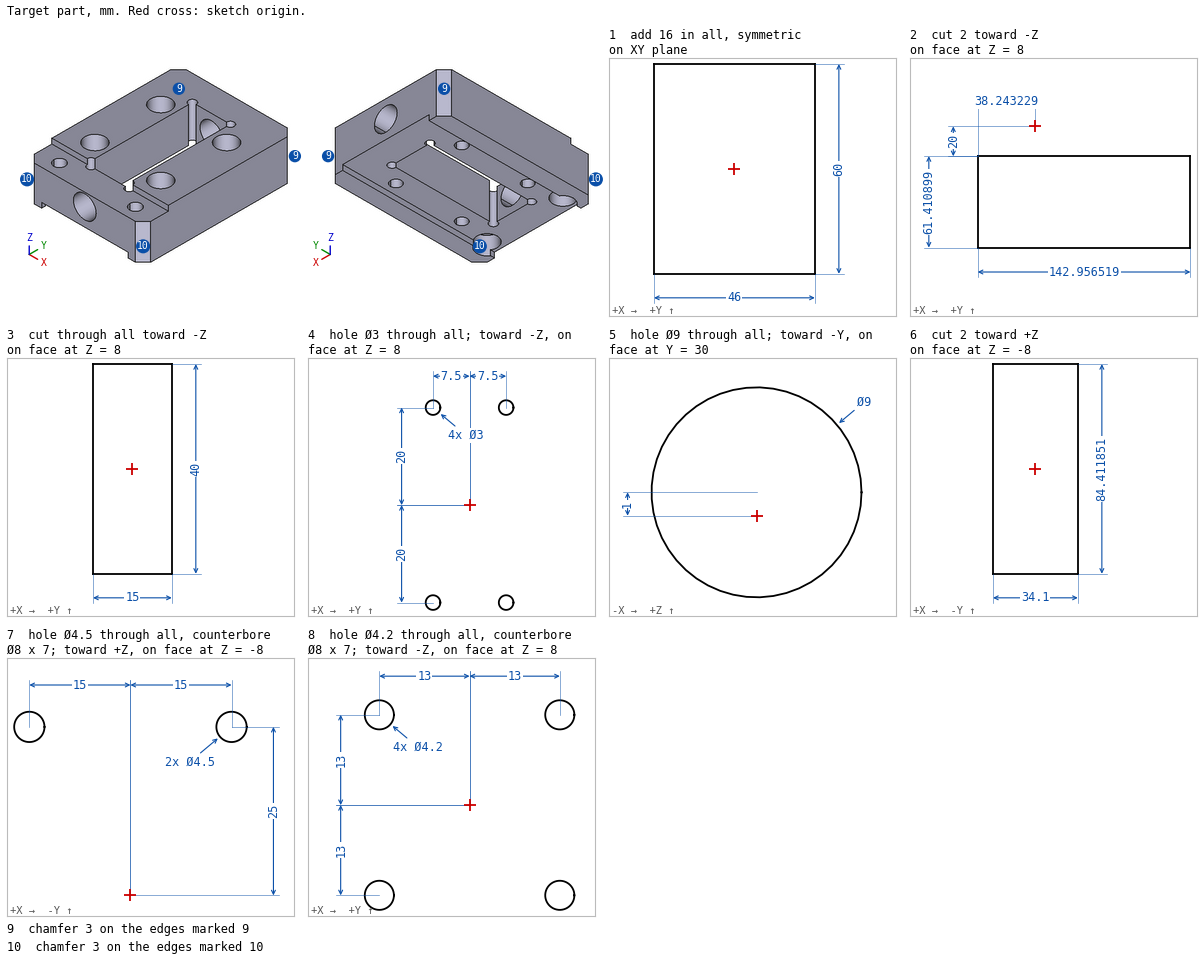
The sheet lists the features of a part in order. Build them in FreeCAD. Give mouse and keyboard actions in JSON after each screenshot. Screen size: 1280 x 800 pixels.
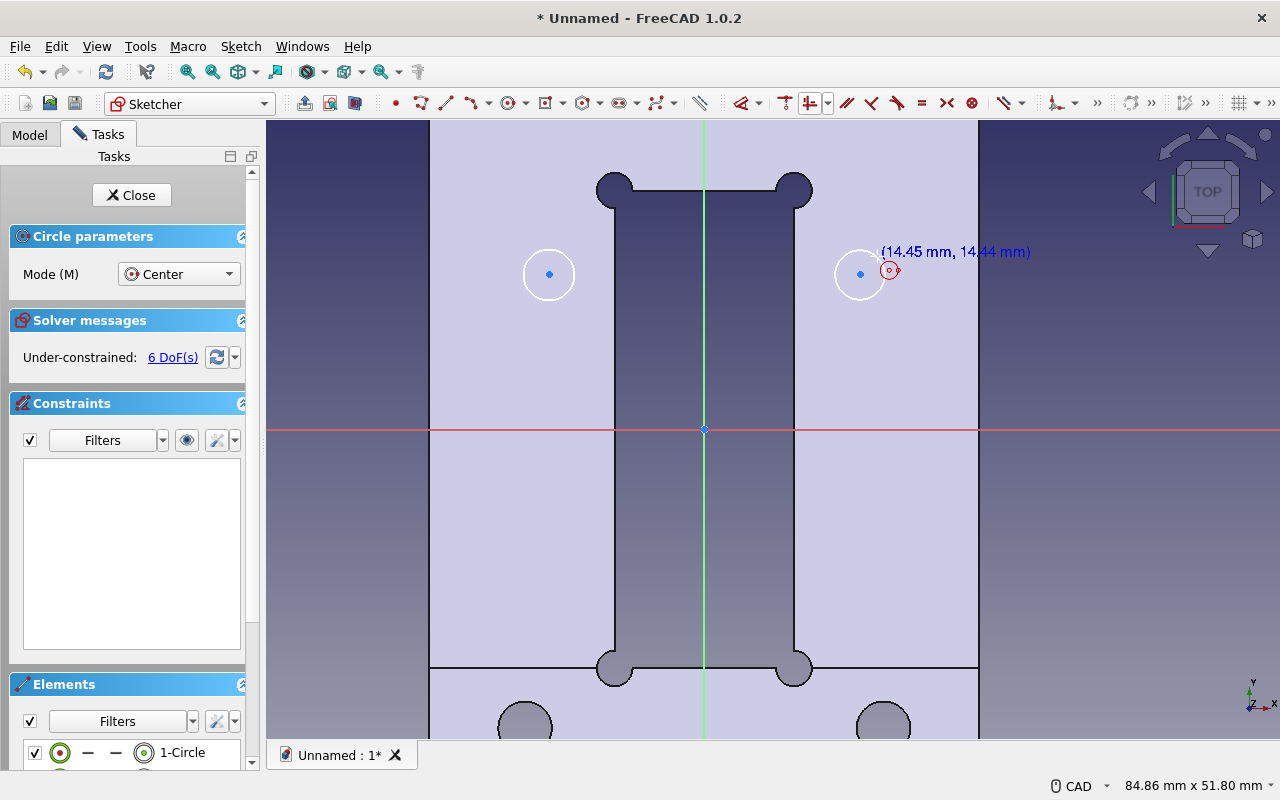
{"action": "left_click", "coordinate": [549, 585]}
{"action": "left_click", "coordinate": [567, 567]}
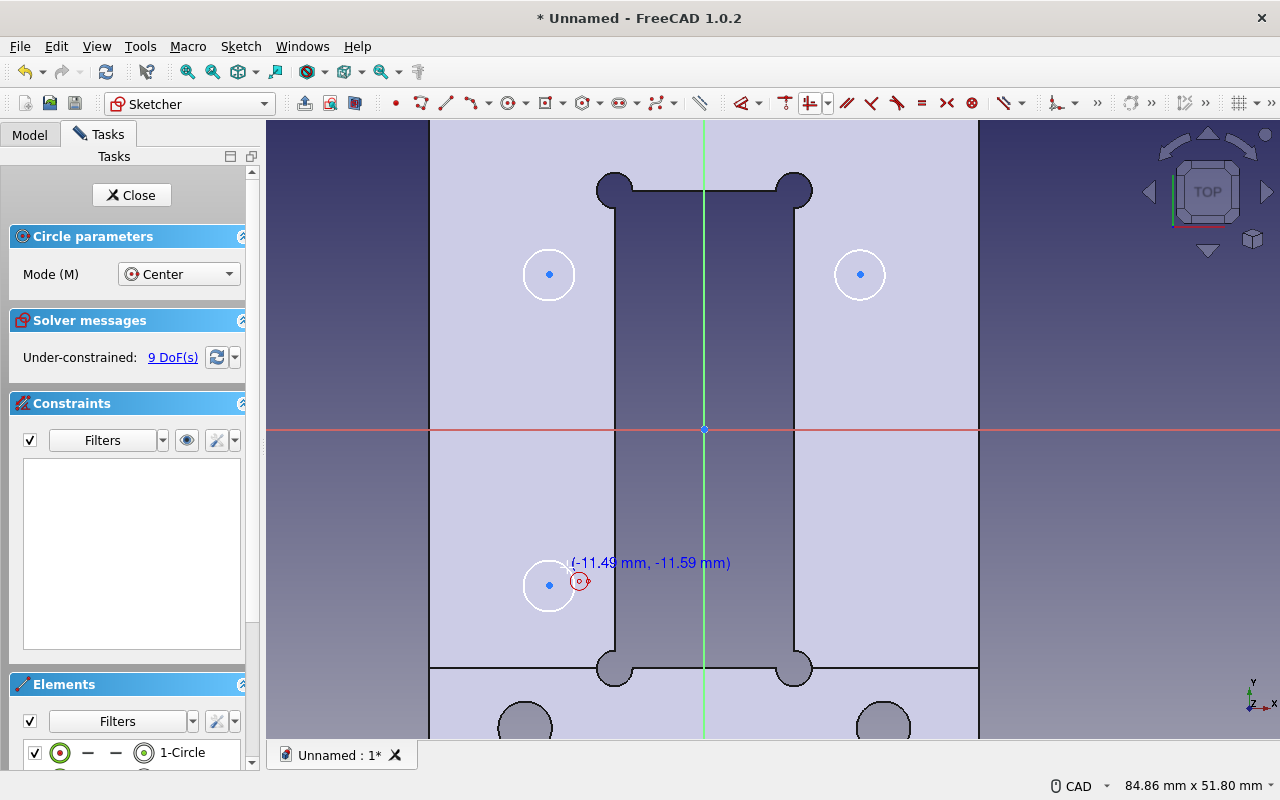
{"action": "left_click", "coordinate": [860, 585]}
{"action": "left_click", "coordinate": [877, 567]}
{"action": "key", "text": "Escape"}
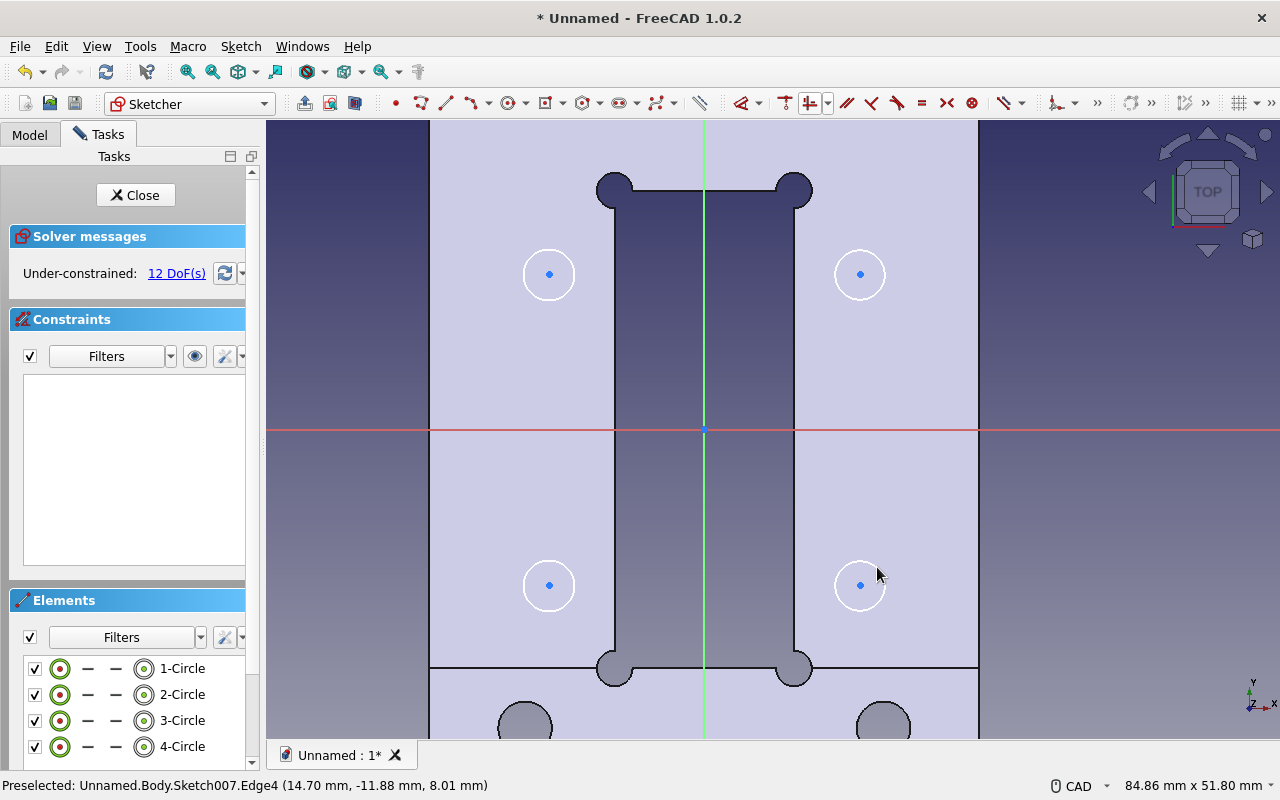
{"action": "left_click", "coordinate": [567, 257]}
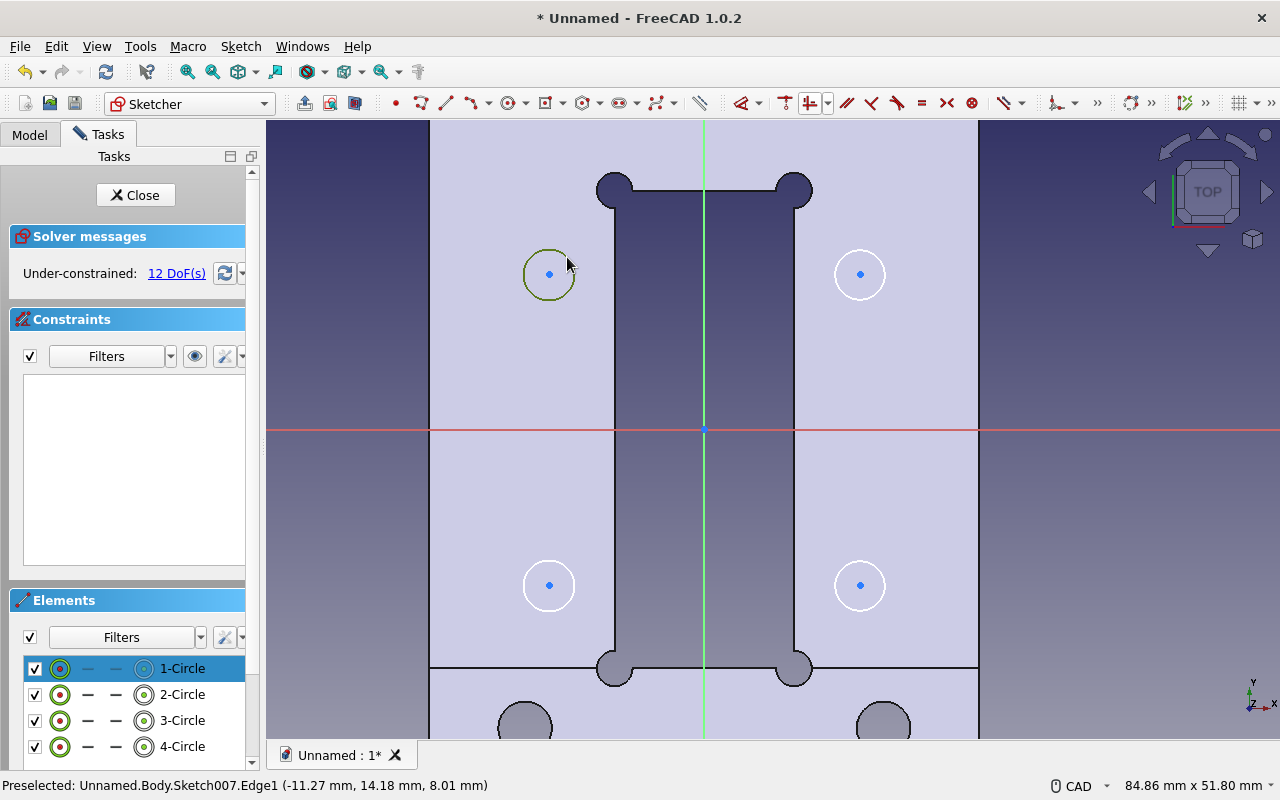
{"action": "left_click", "coordinate": [877, 257]}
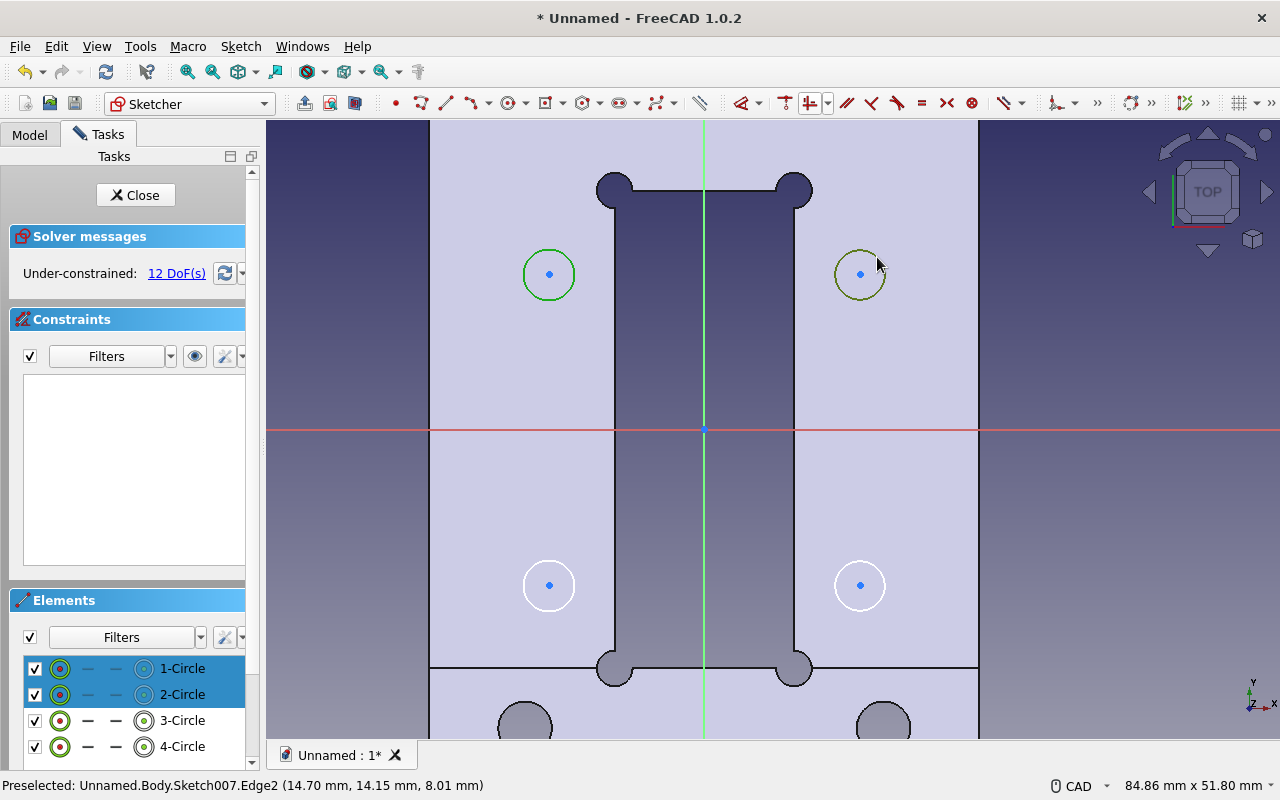
{"action": "left_click", "coordinate": [567, 568]}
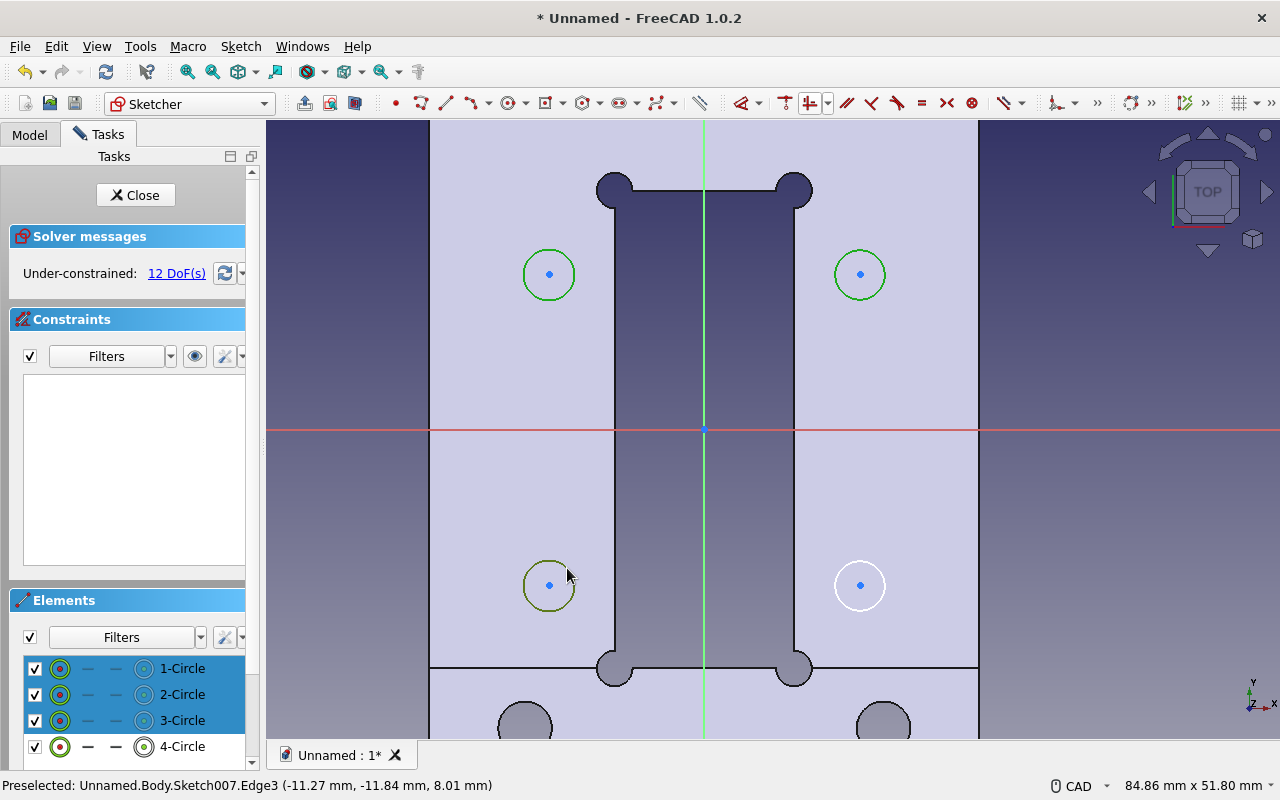
{"action": "left_click", "coordinate": [877, 568]}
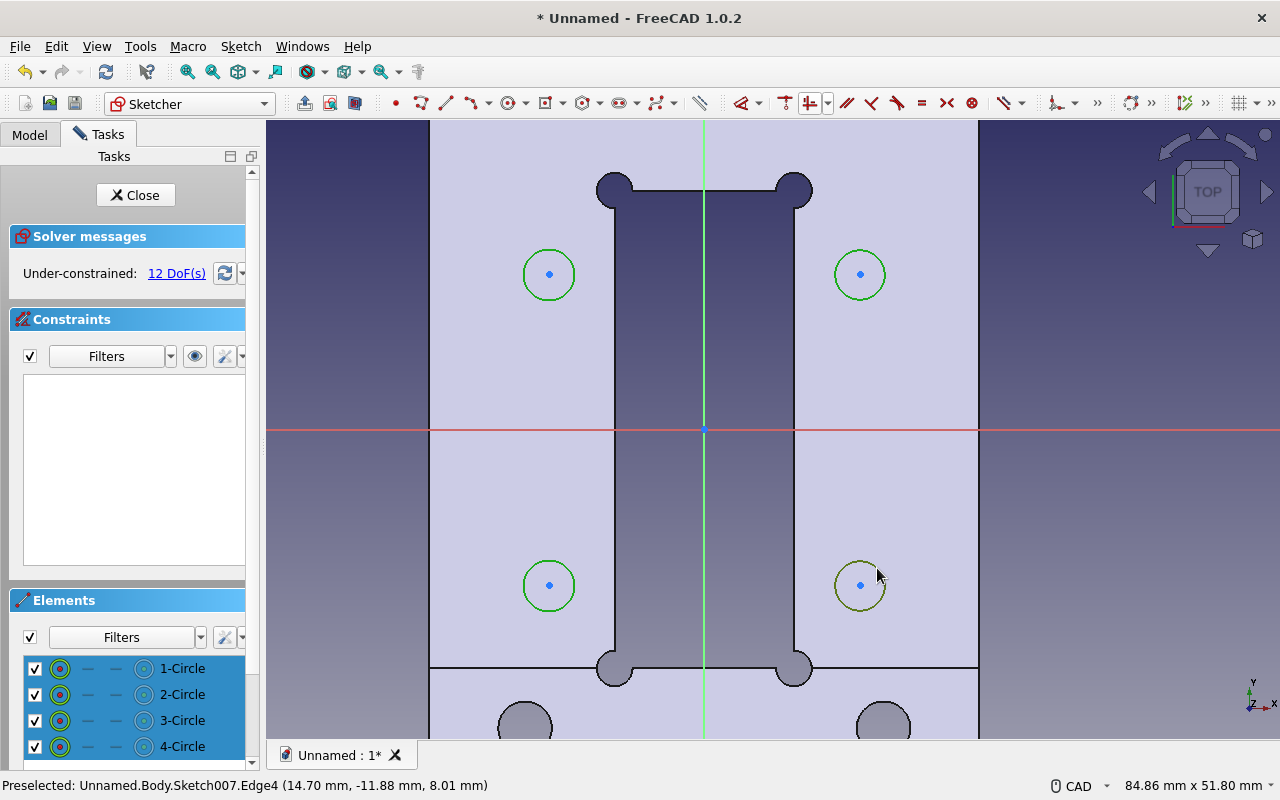
{"action": "left_click", "coordinate": [922, 104]}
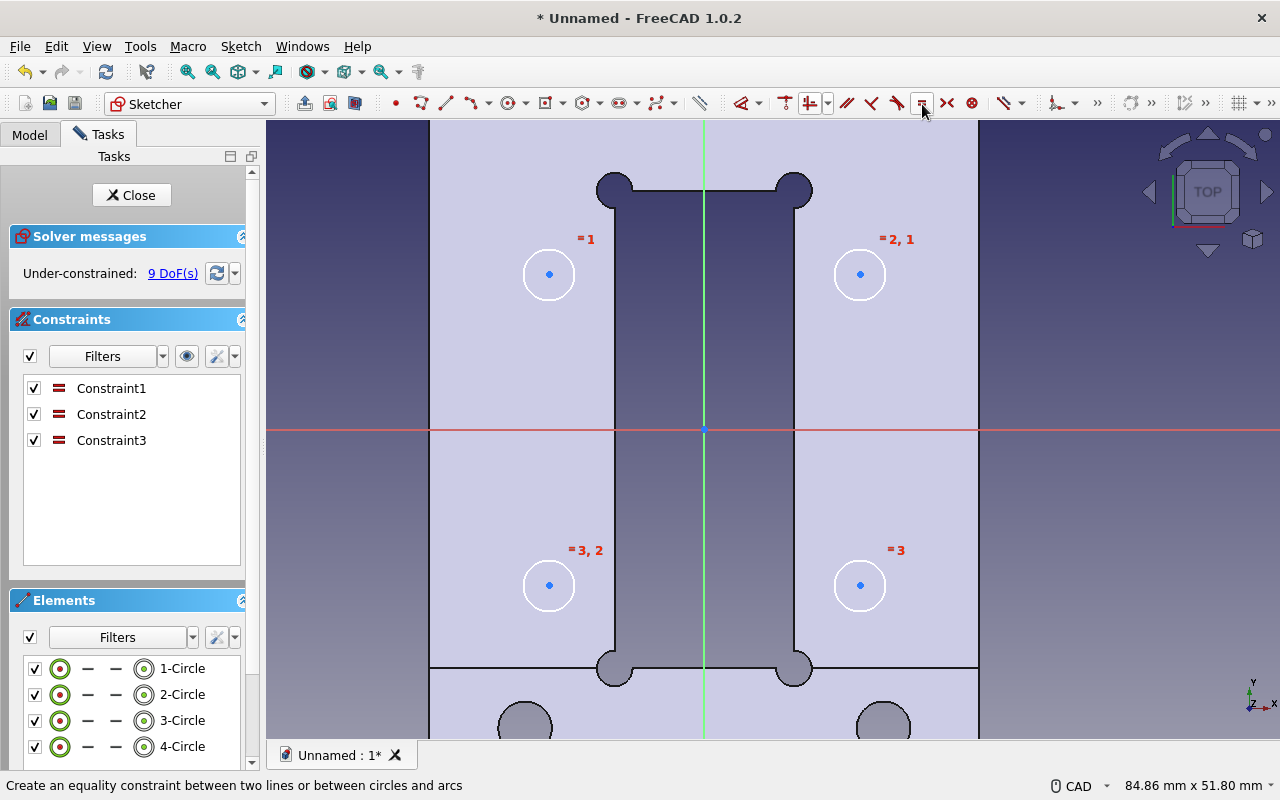
{"action": "left_click", "coordinate": [549, 275]}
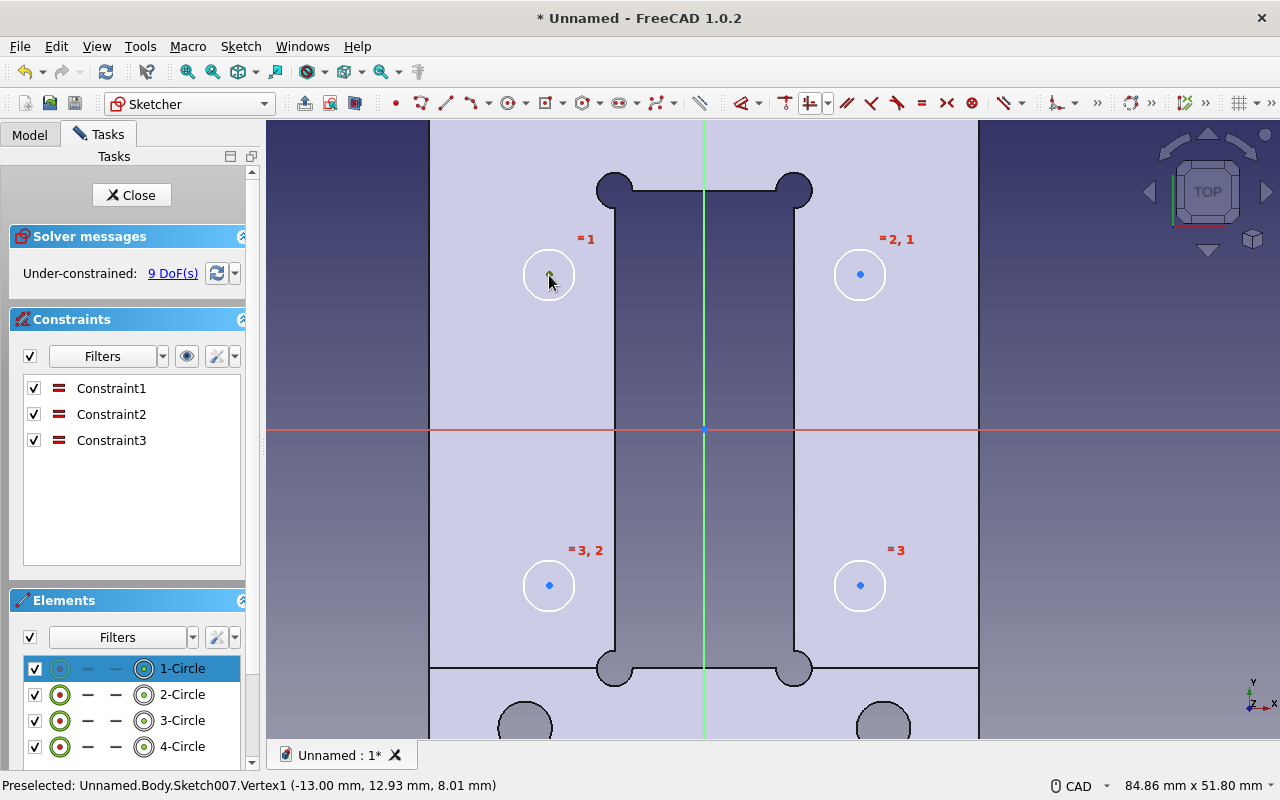
{"action": "left_click", "coordinate": [860, 275]}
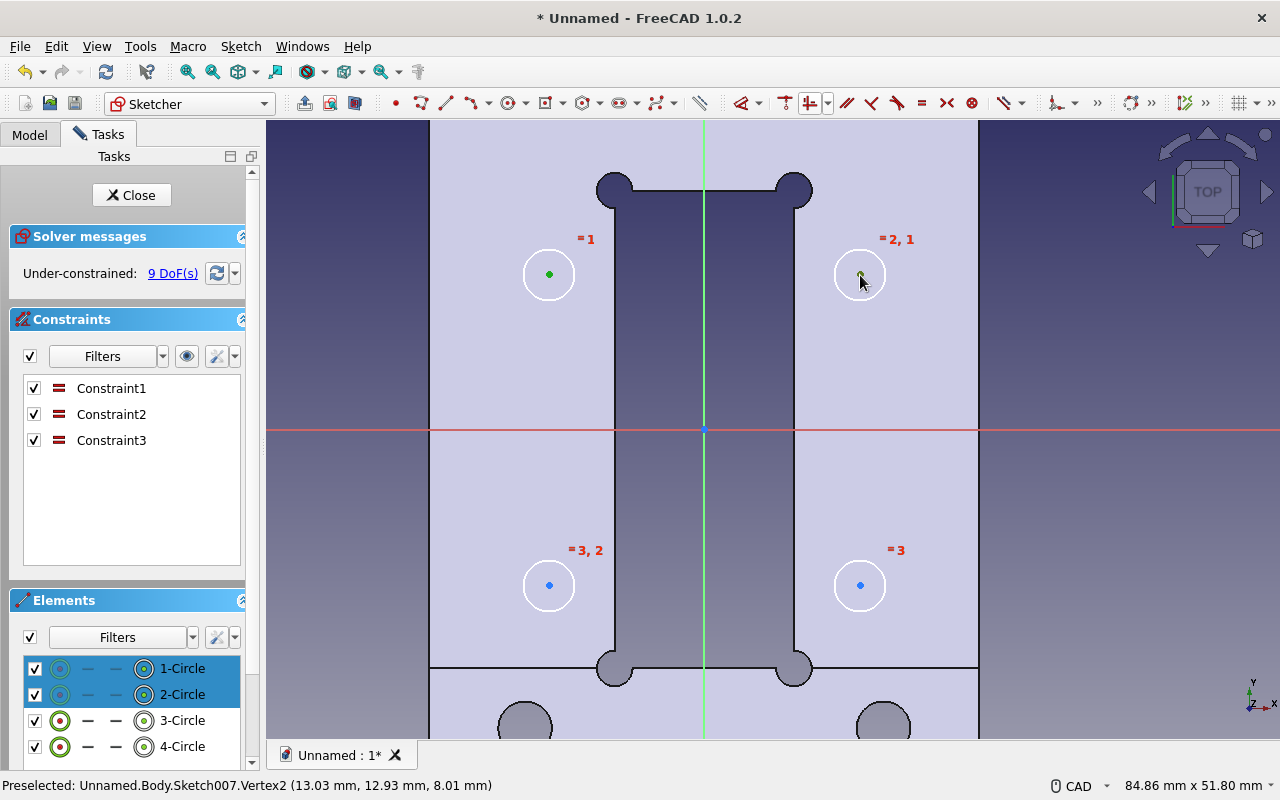
{"action": "key", "text": "h"}